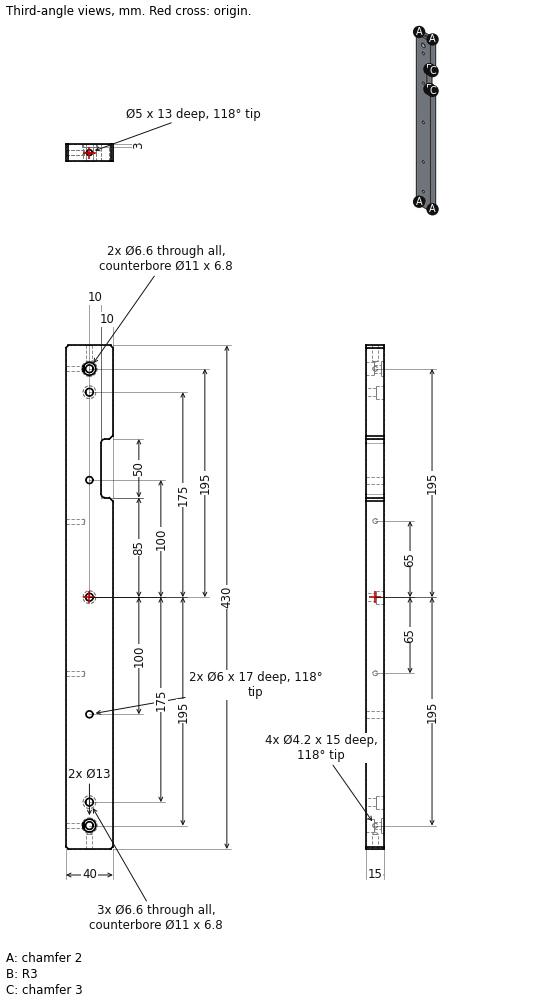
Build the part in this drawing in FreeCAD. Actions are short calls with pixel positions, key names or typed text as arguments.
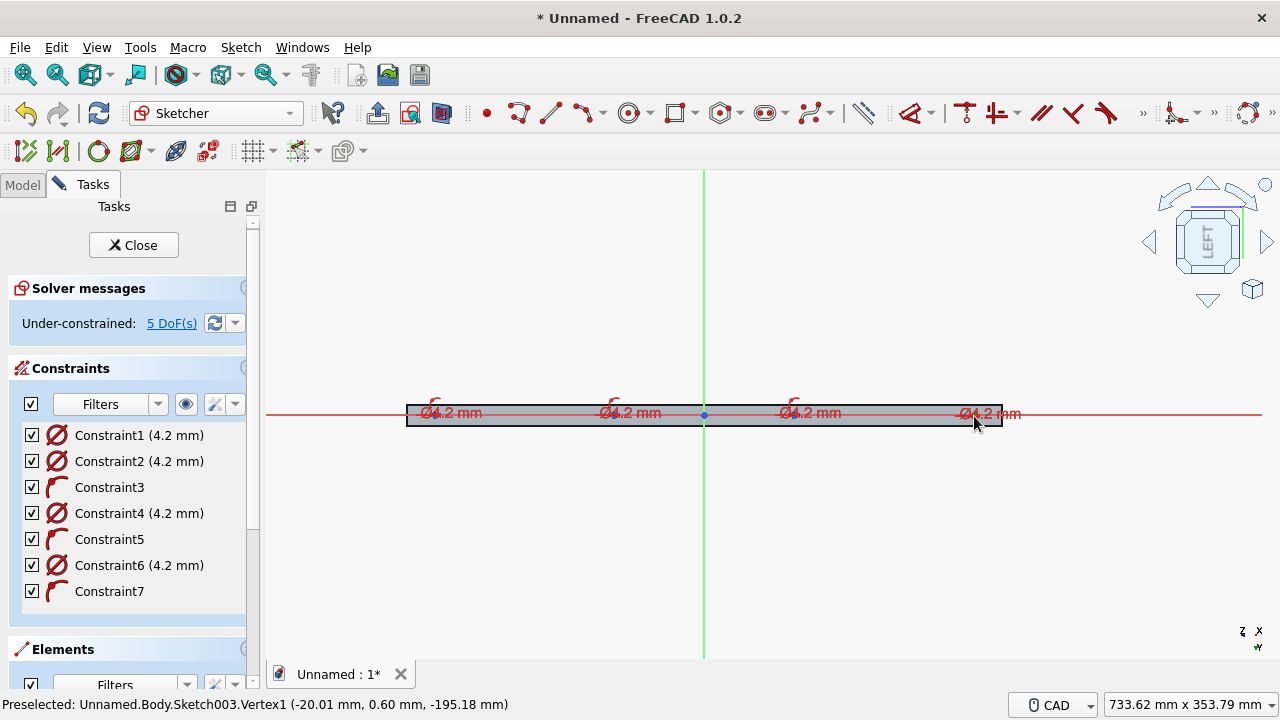
click(353, 415)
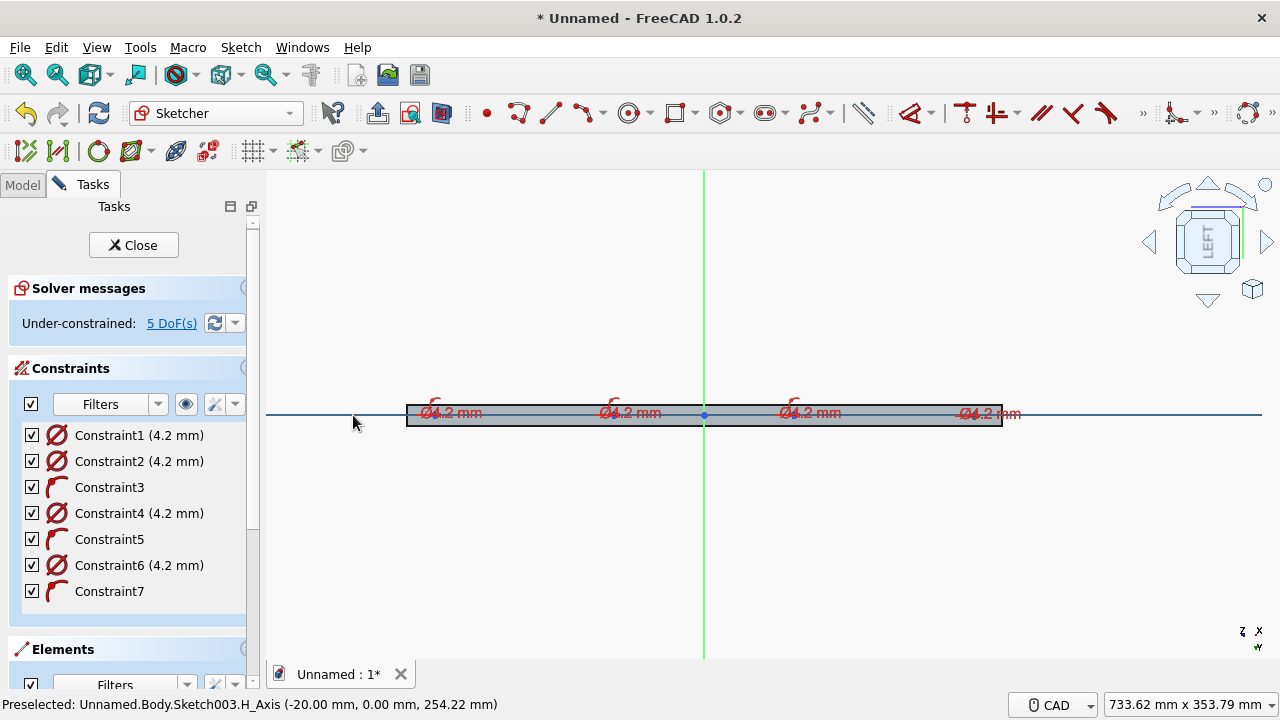
click(966, 114)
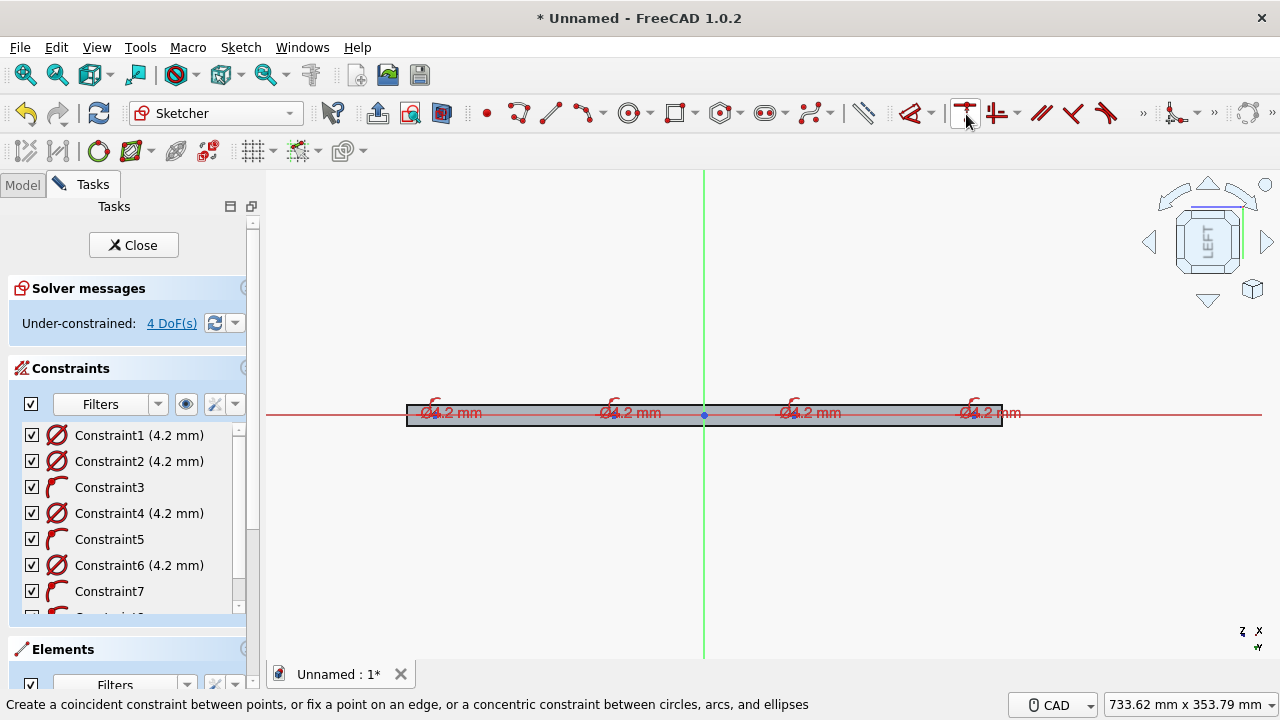
click(910, 114)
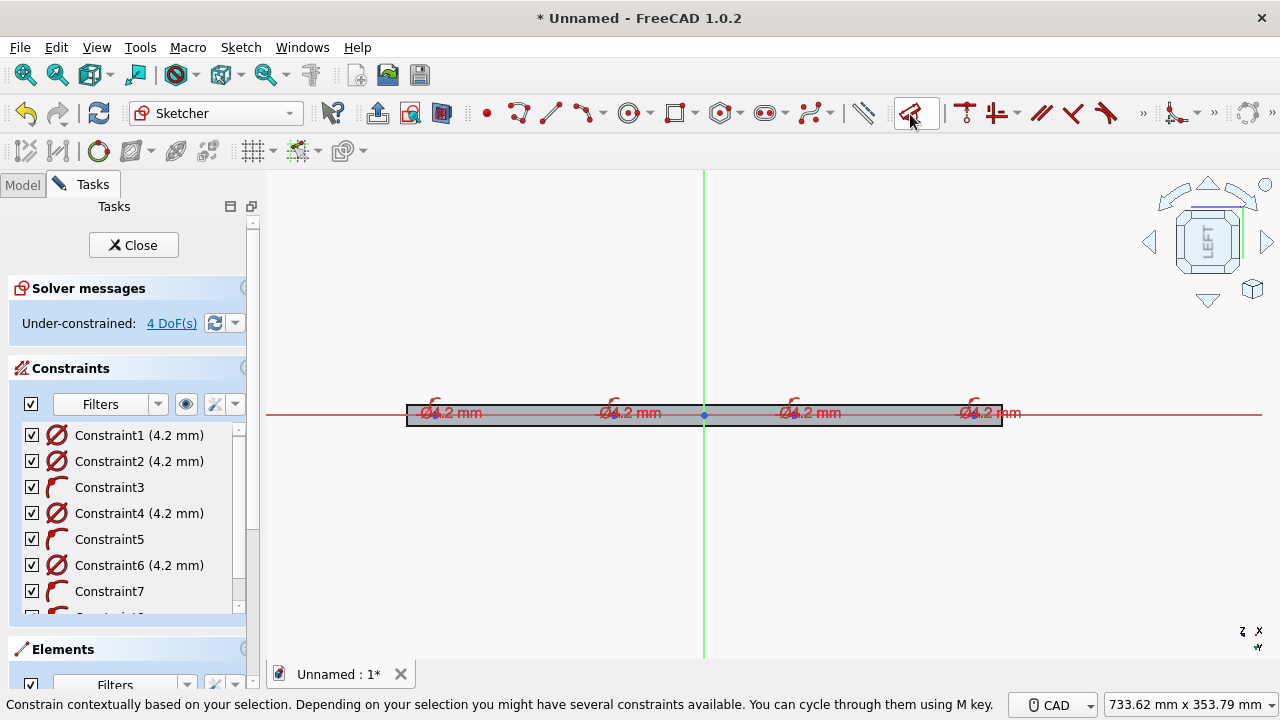
click(794, 415)
click(749, 449)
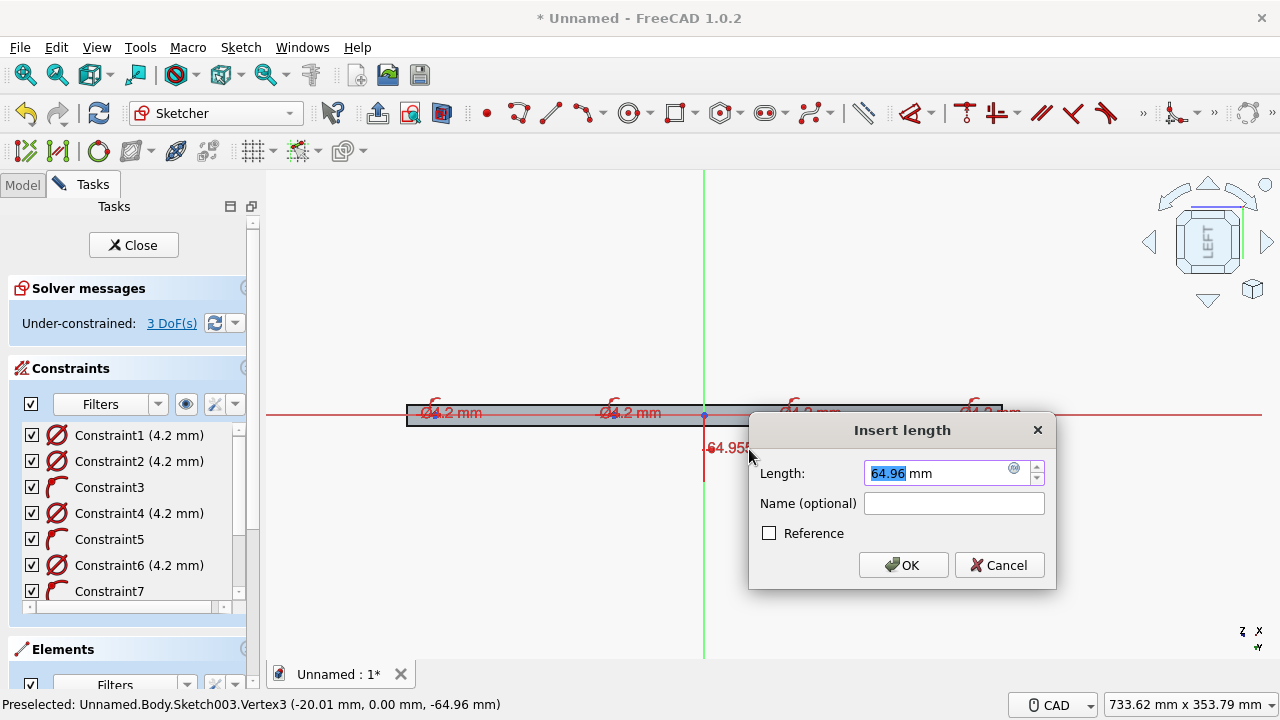
text(65)
key(Return)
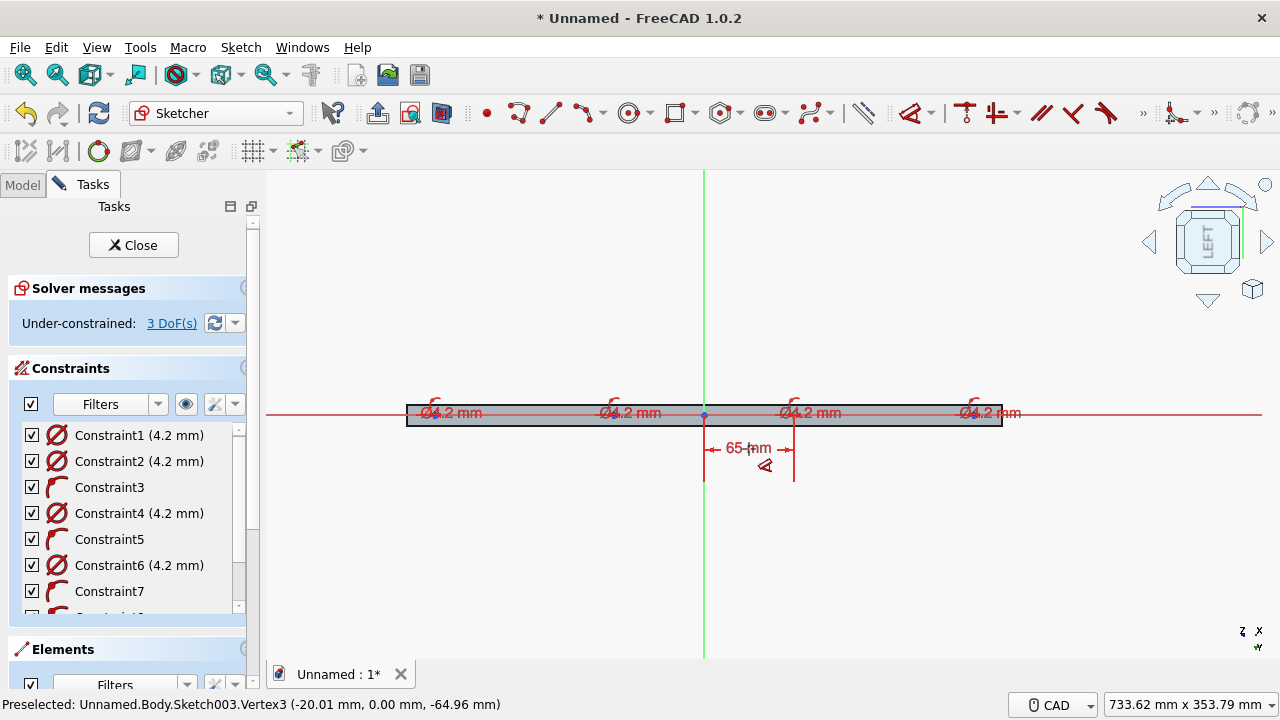
click(614, 415)
click(659, 449)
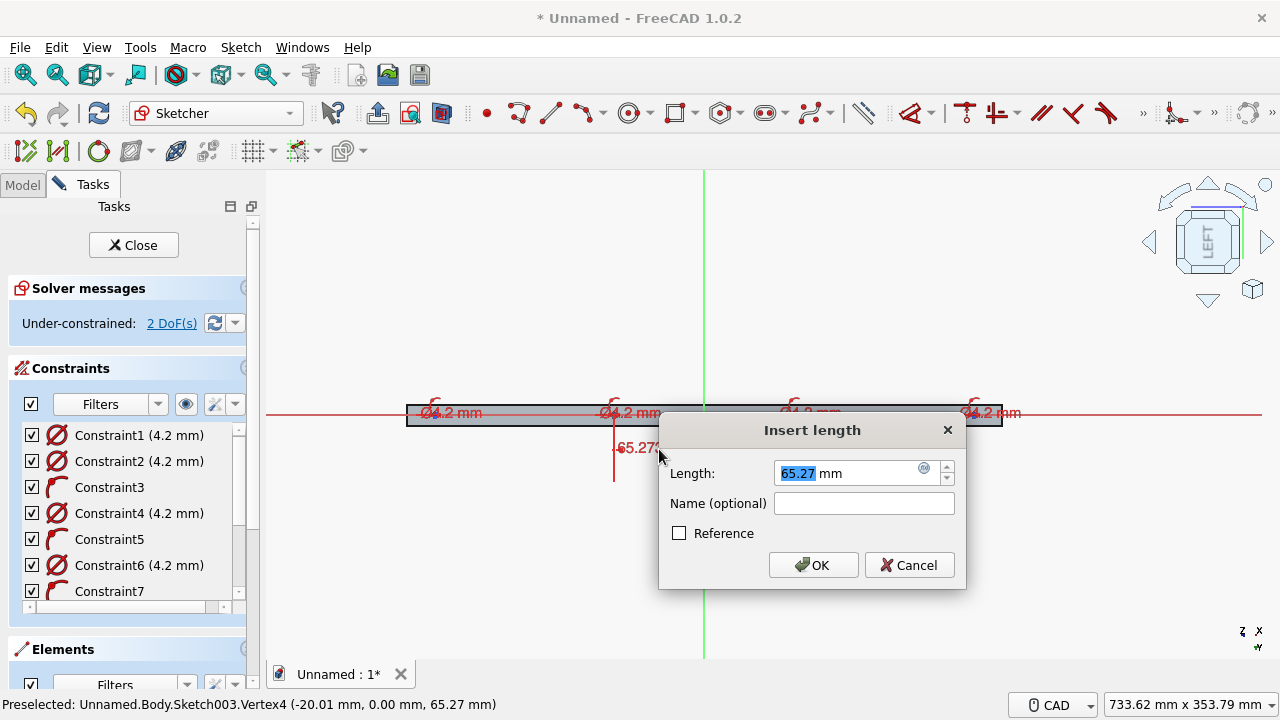
text(65)
key(Return)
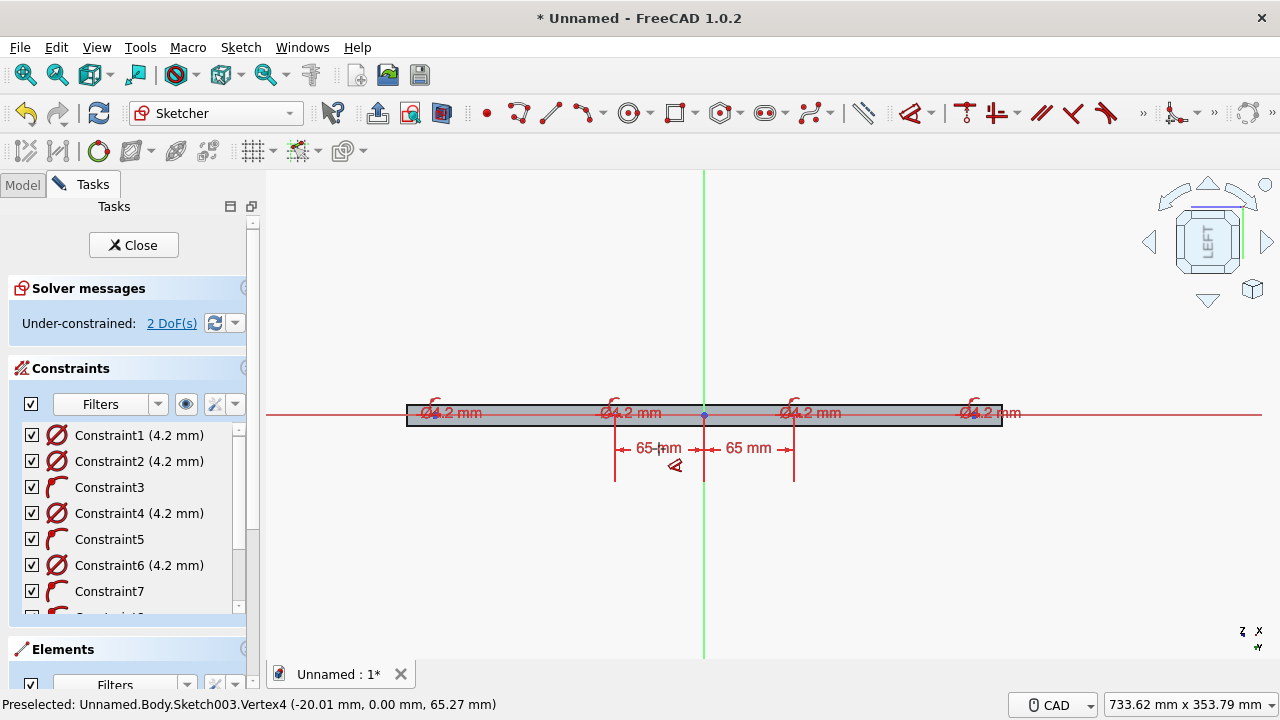
click(974, 415)
click(839, 449)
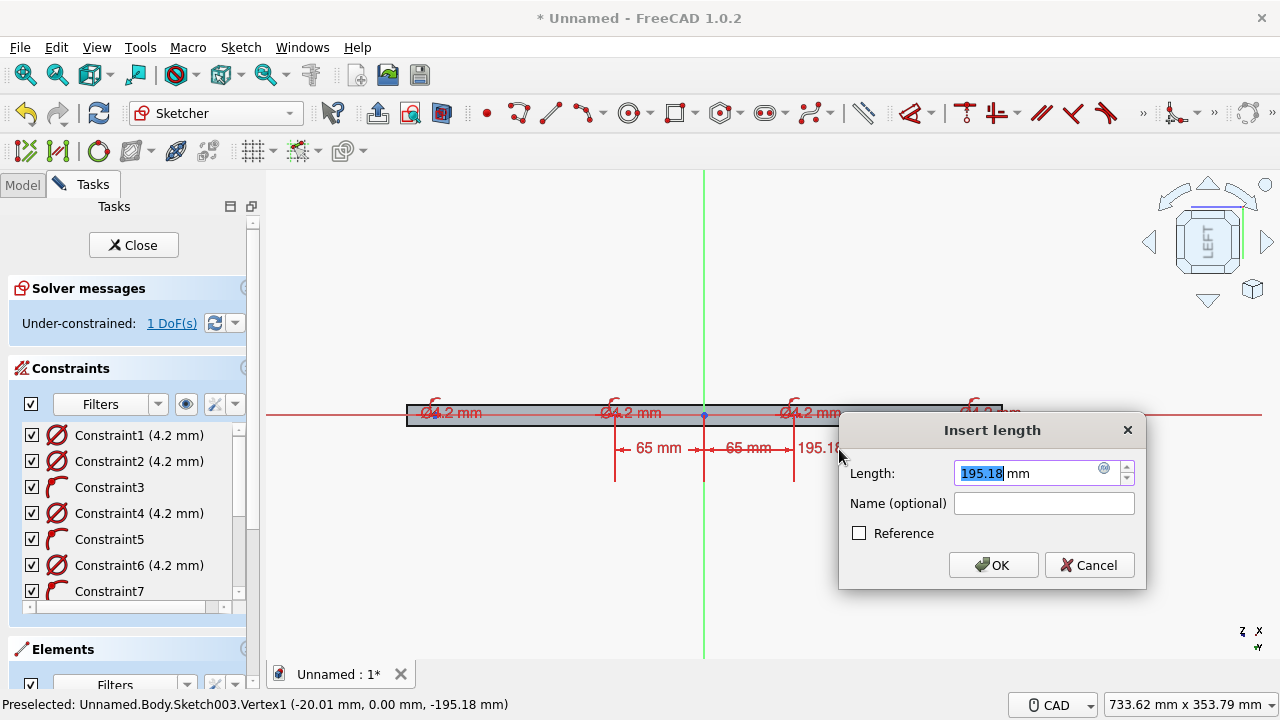
text(195)
key(Return)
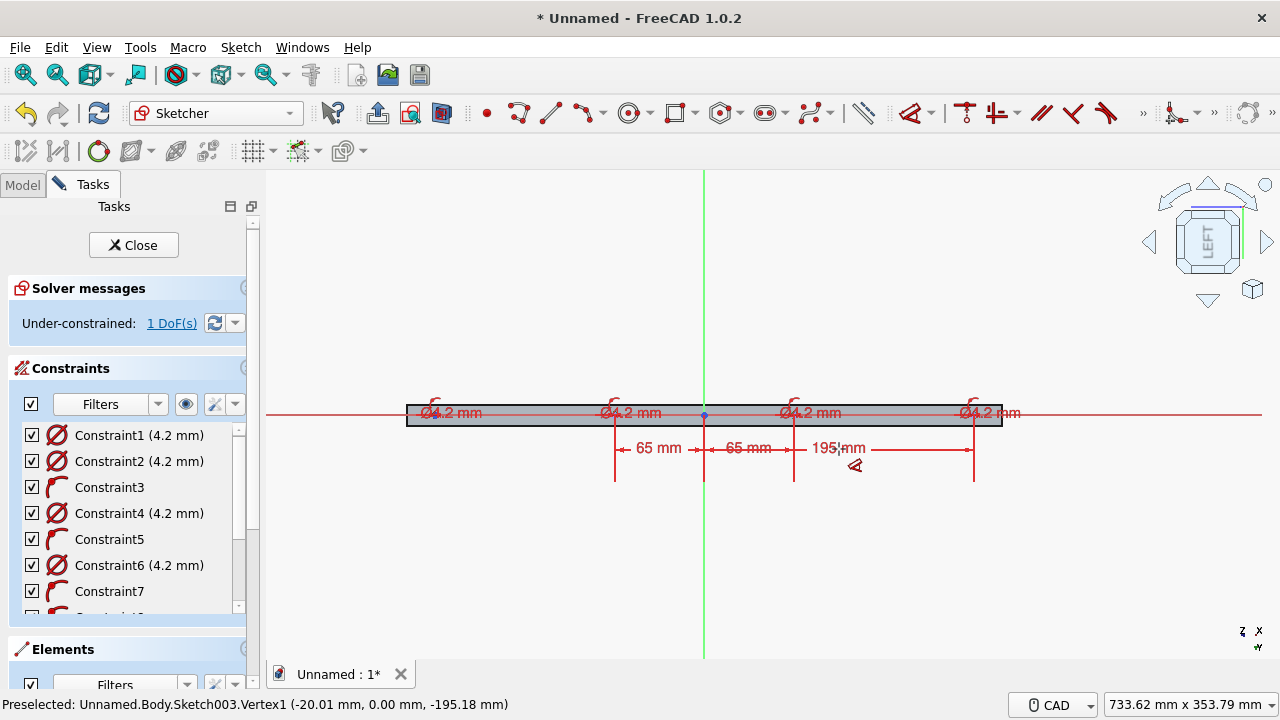
click(435, 415)
click(570, 449)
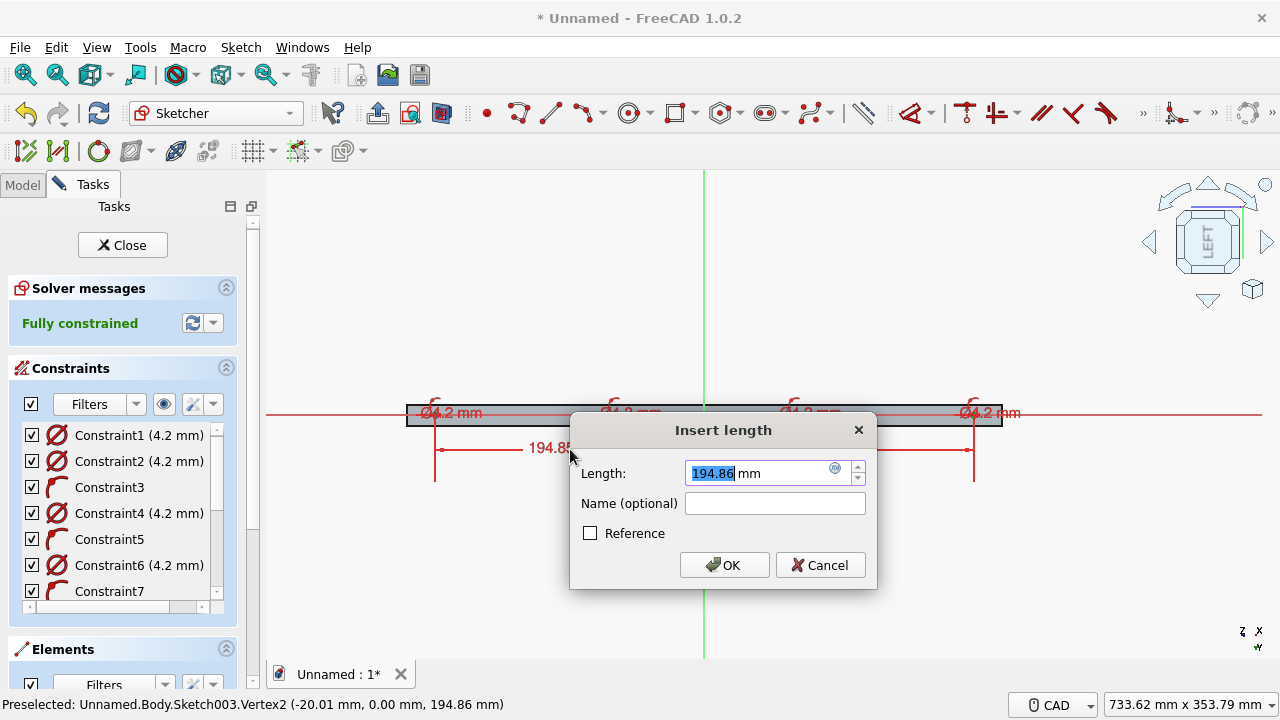
text(195)
key(Return)
key(Escape)